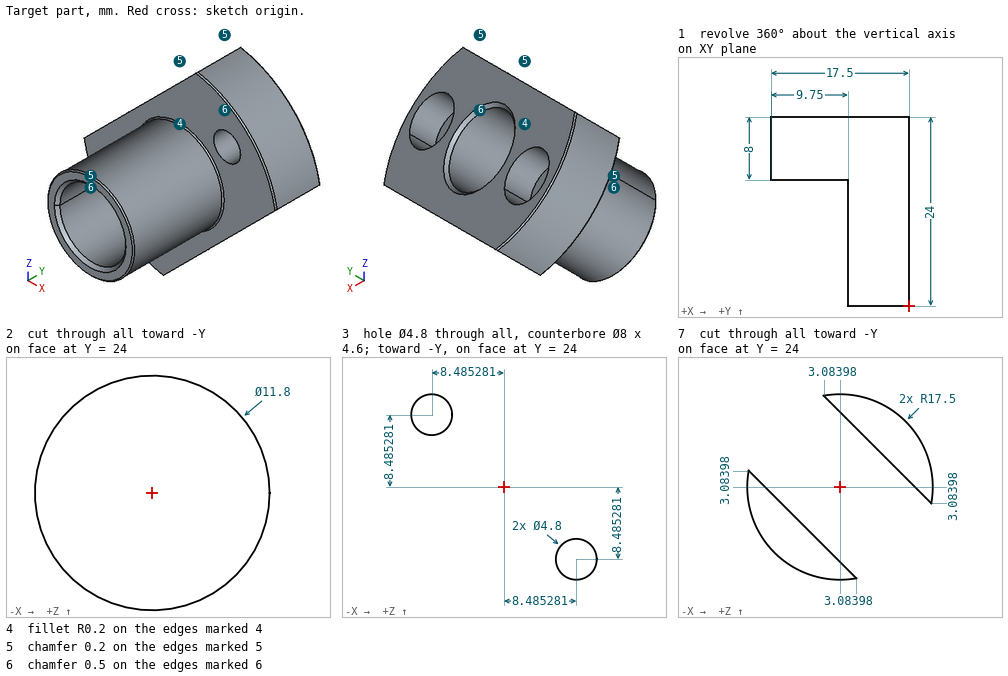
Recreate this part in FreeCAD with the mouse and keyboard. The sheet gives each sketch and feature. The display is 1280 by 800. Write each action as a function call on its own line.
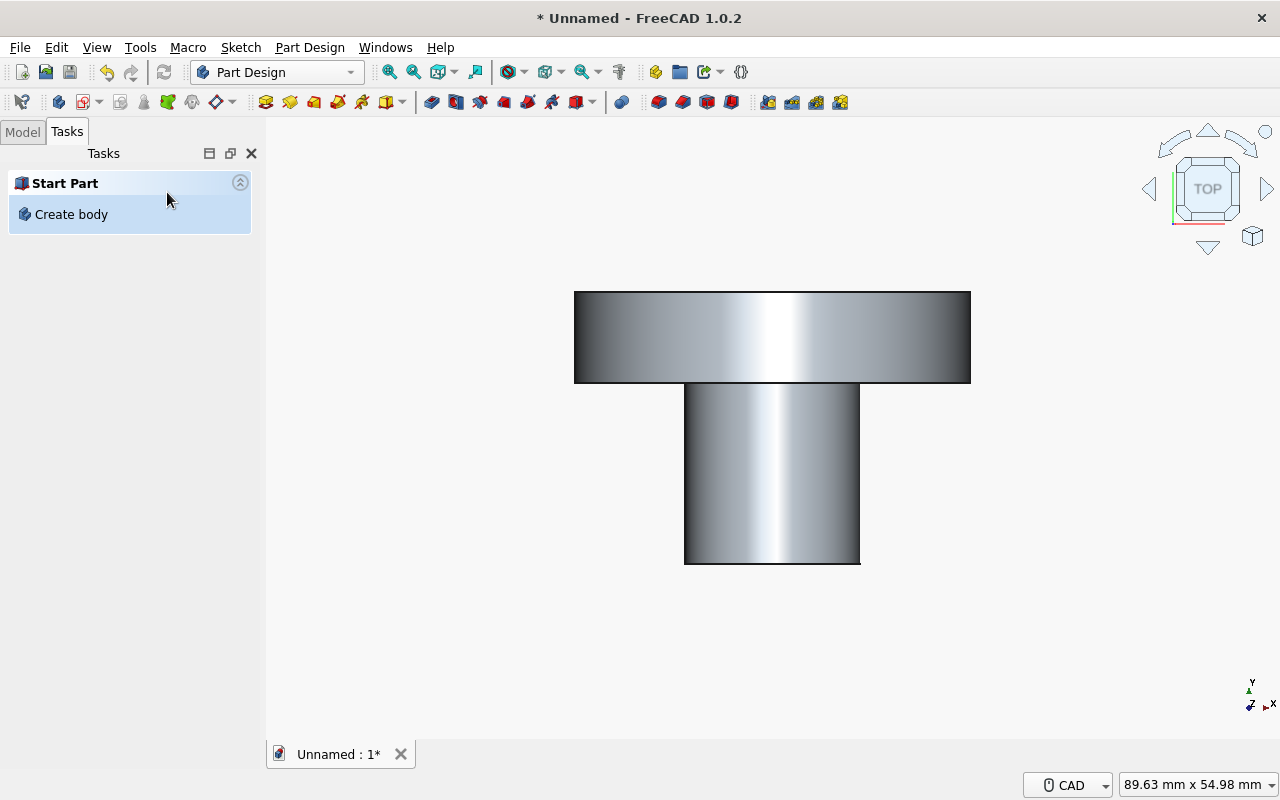
key(v)
key(f)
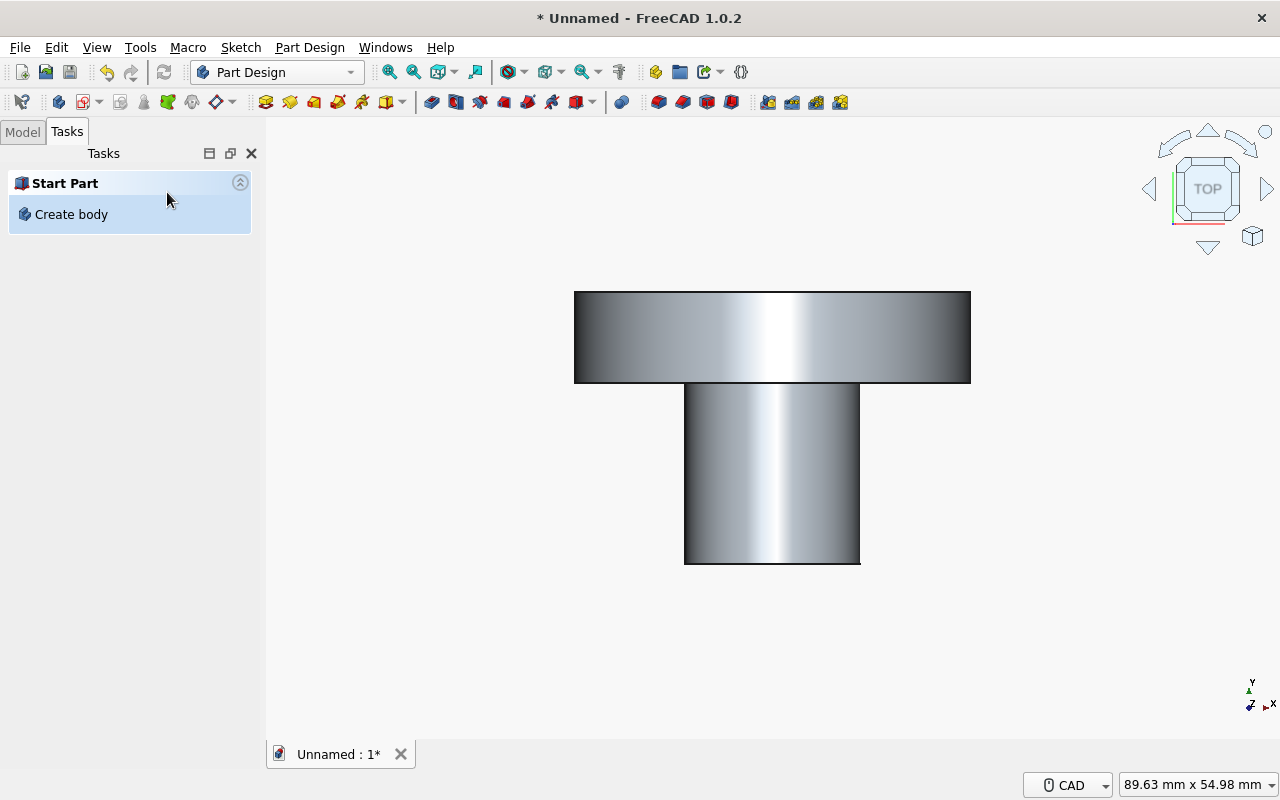
key(1)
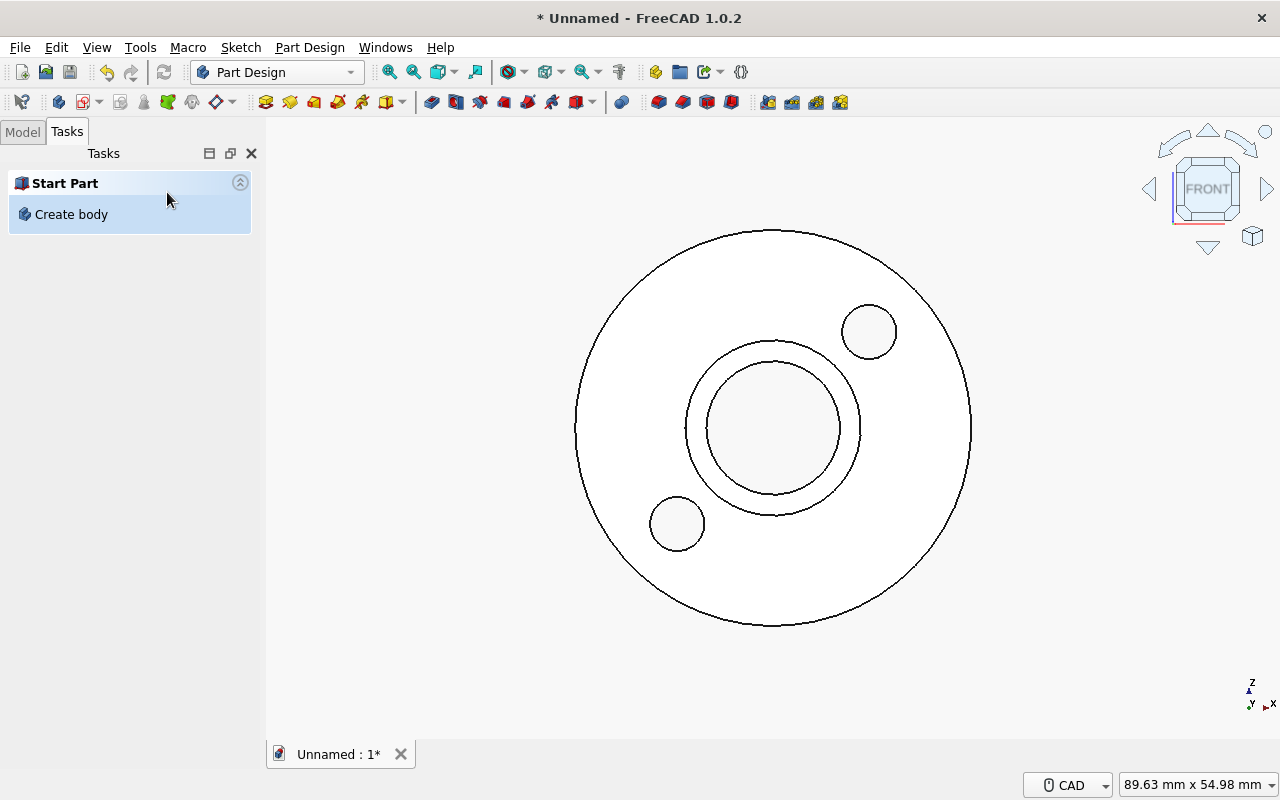
key(3)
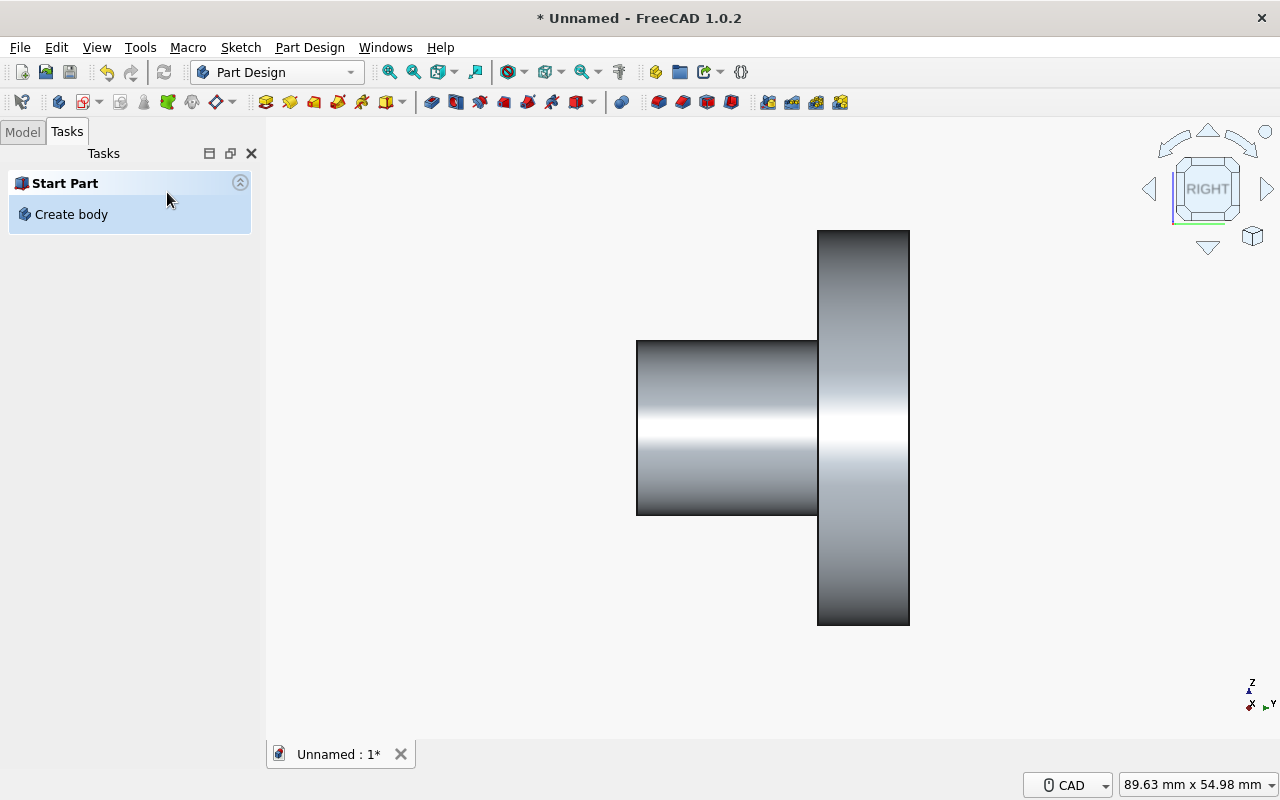
key(5)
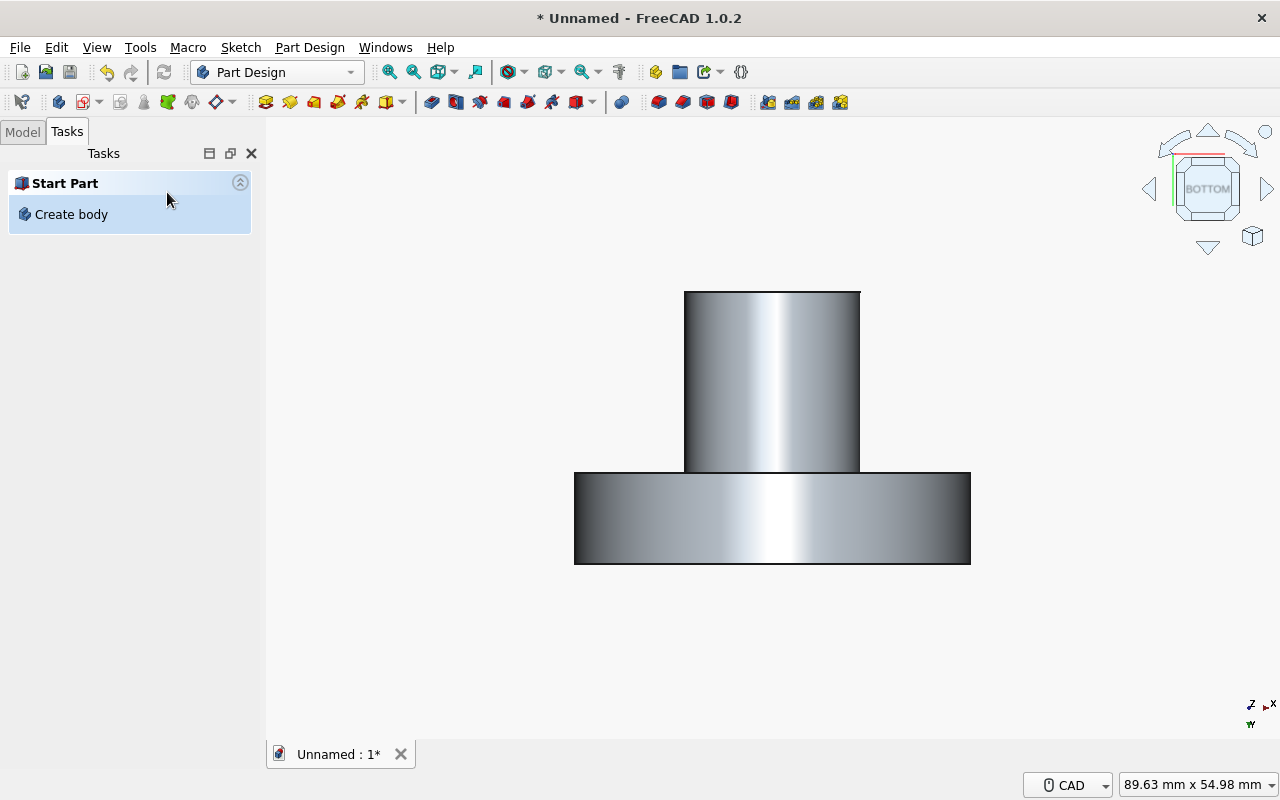
key(v)
key(f)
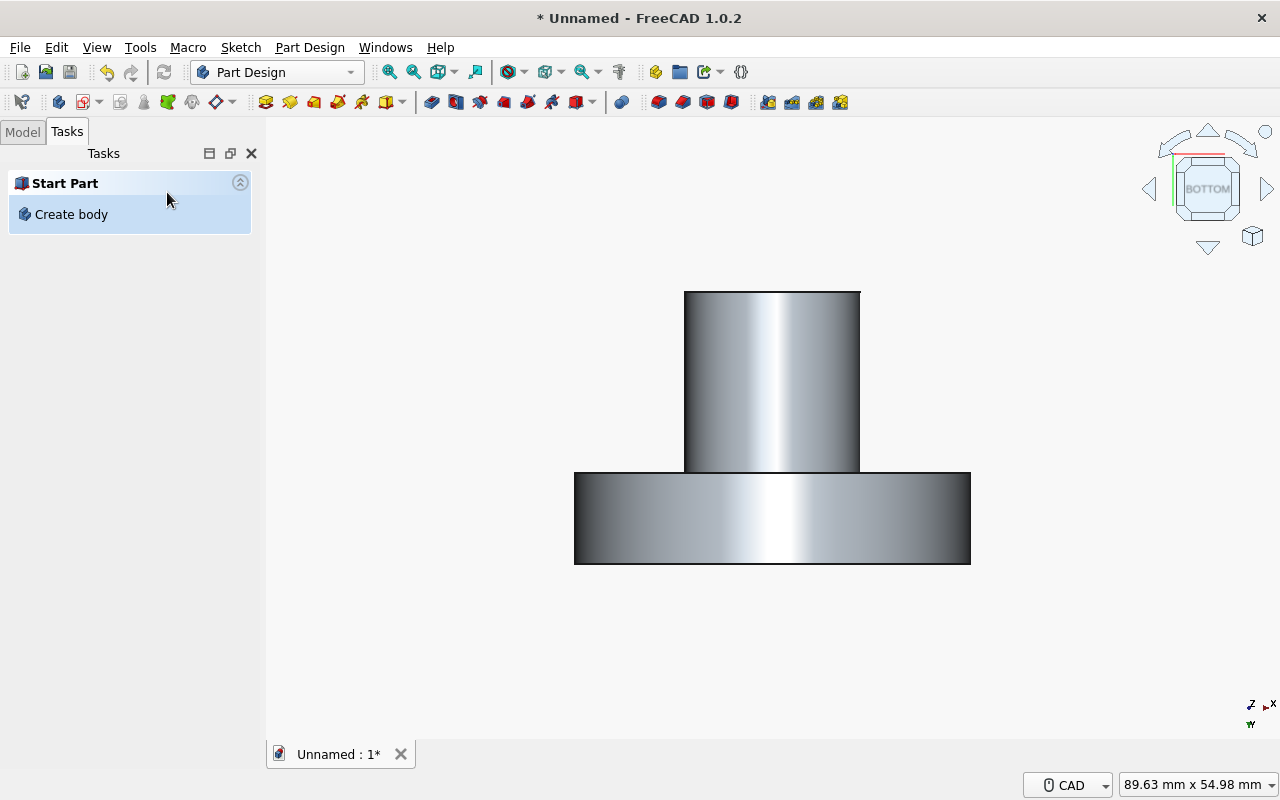
key(4)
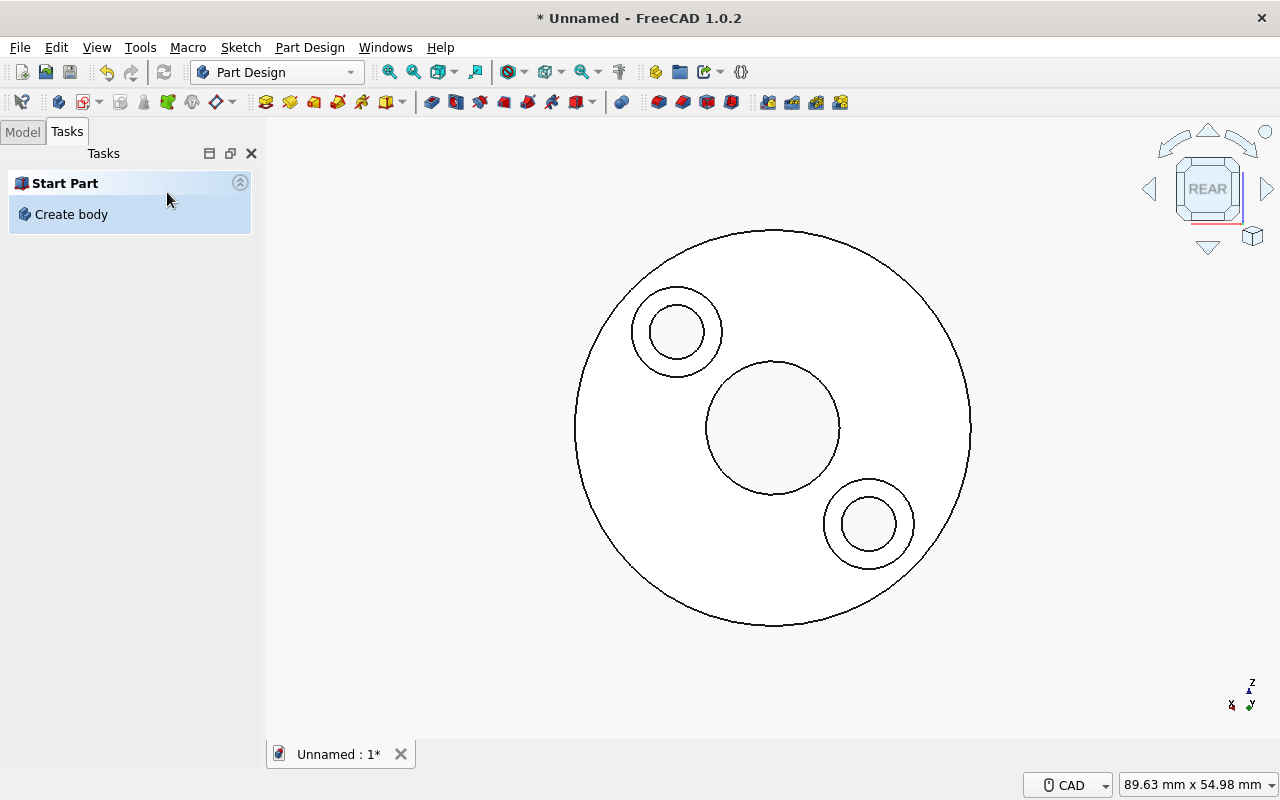
key(6)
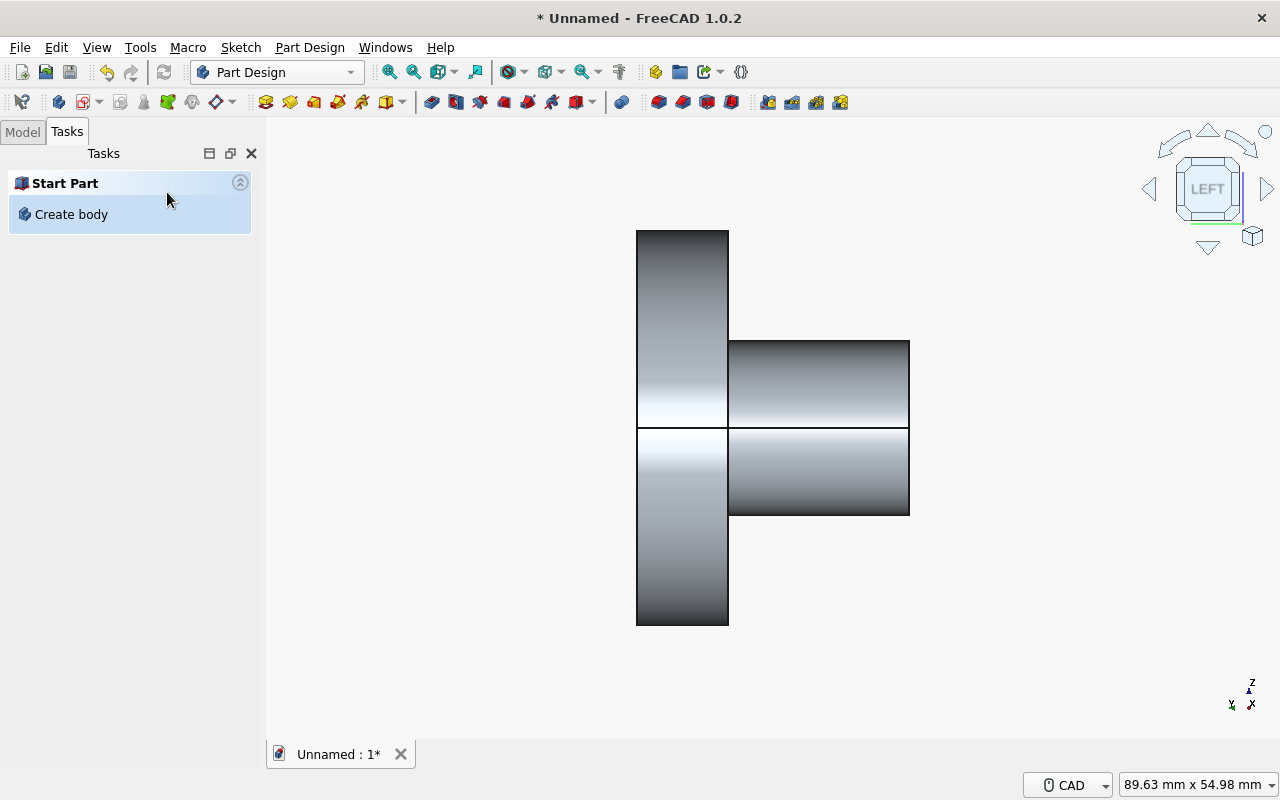
key(v)
key(3)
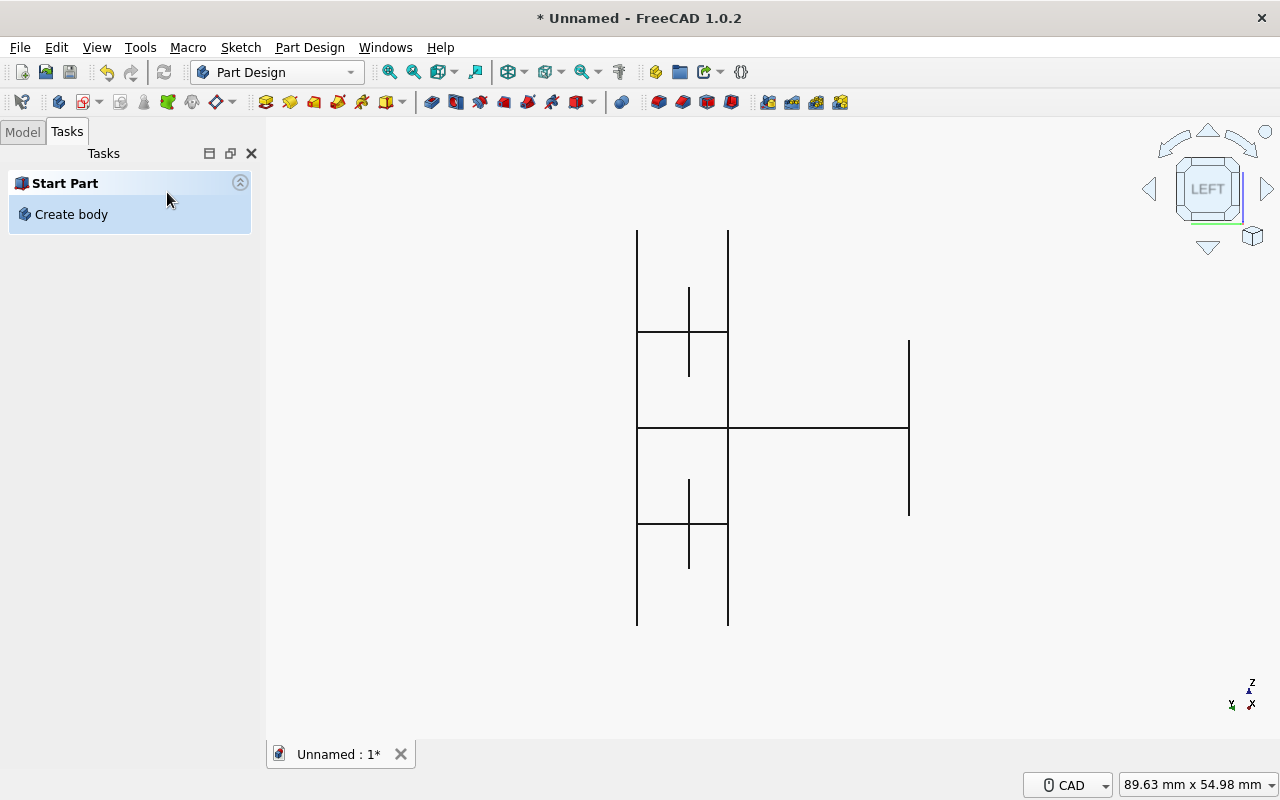
key(0)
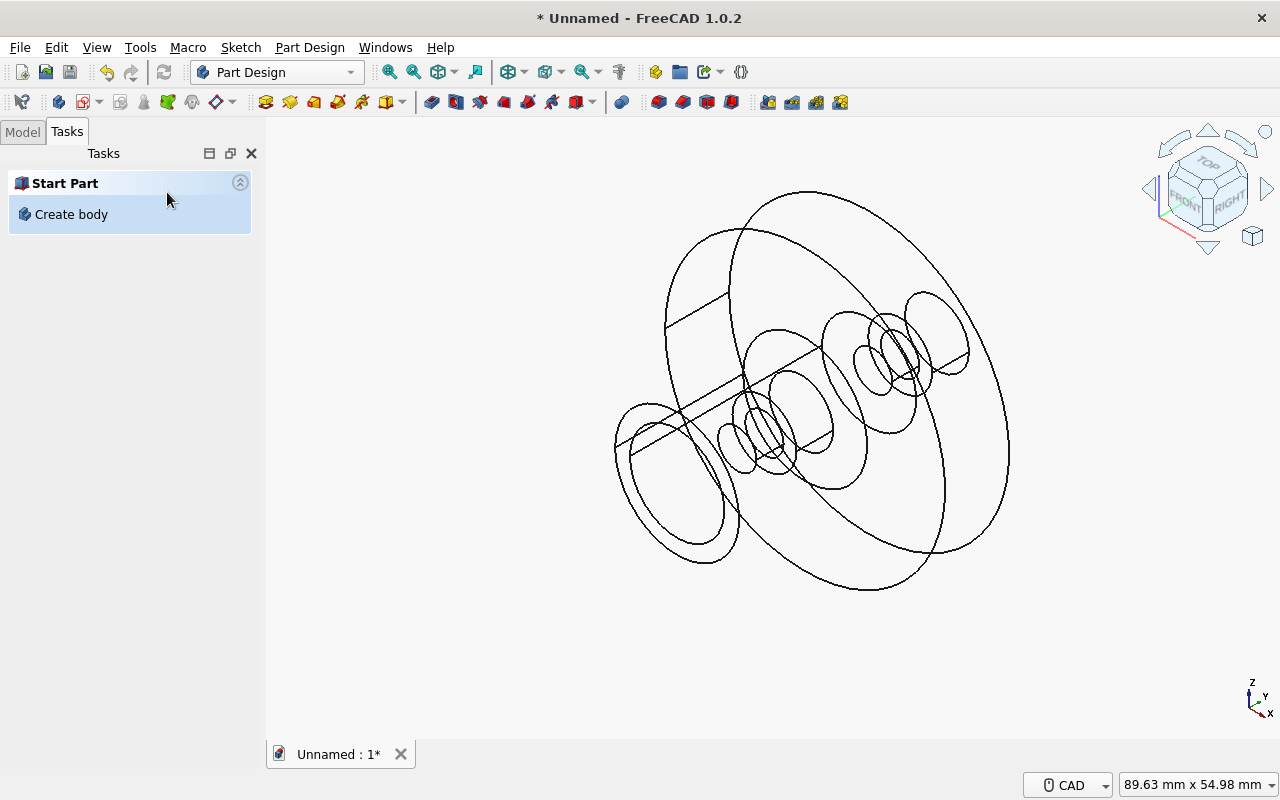
click(867, 444)